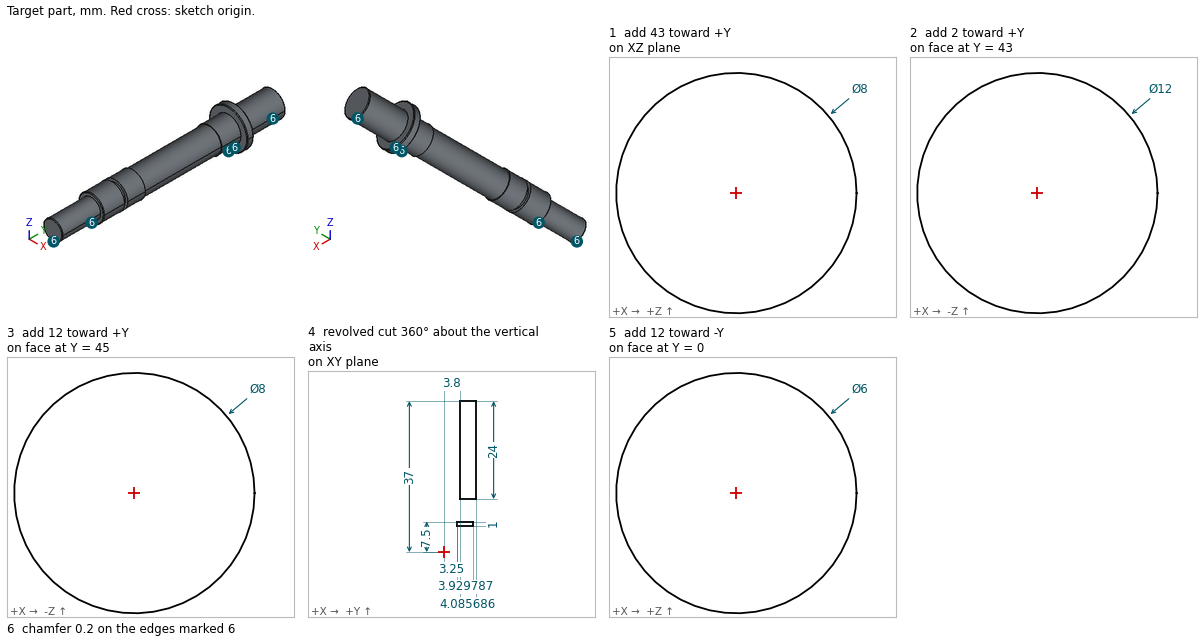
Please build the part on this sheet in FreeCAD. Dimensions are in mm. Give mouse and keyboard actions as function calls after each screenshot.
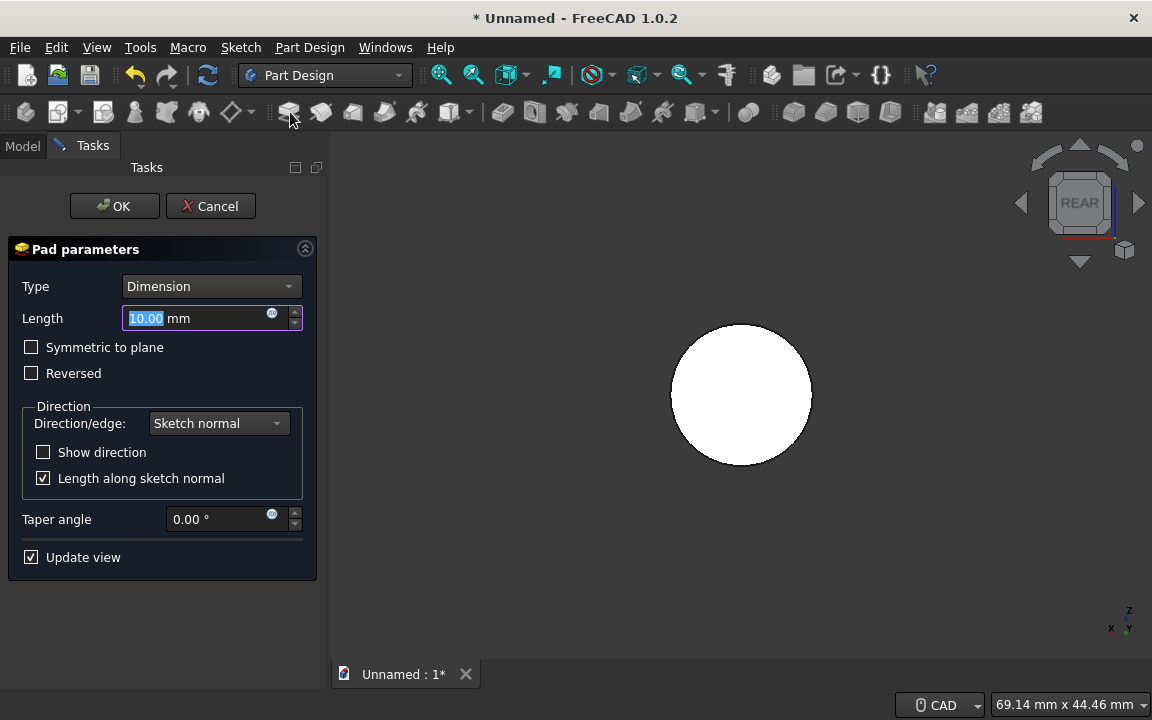
text(2)
key(Tab)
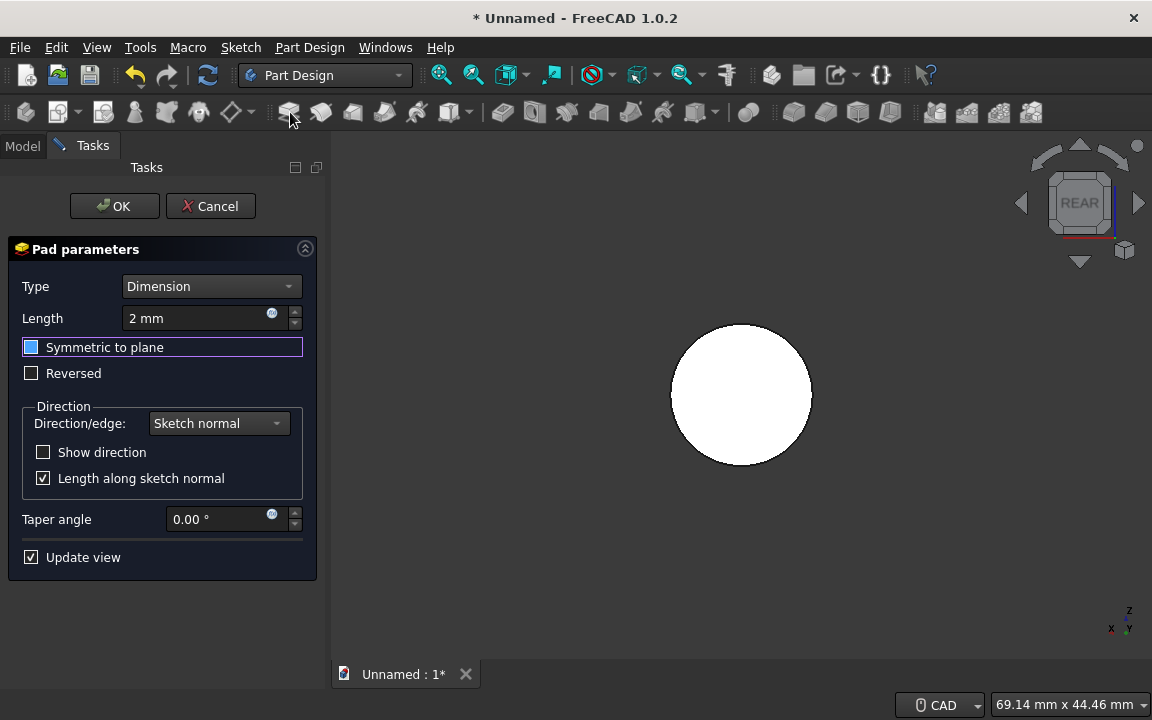
click(115, 206)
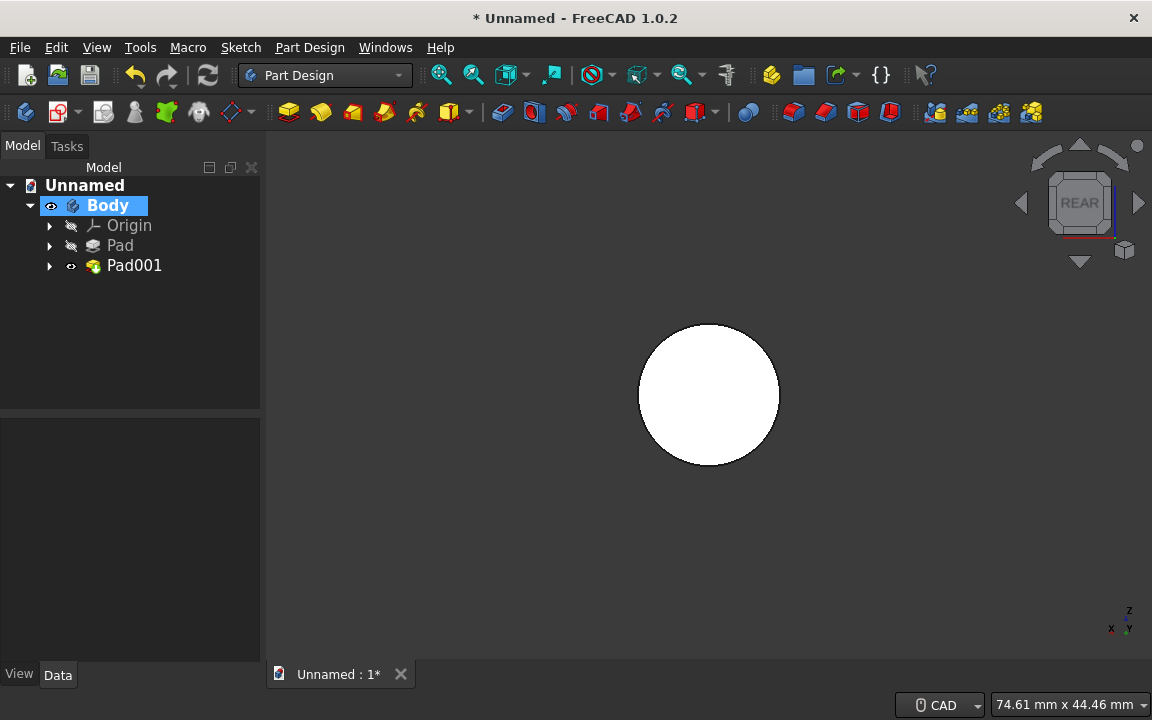
click(442, 76)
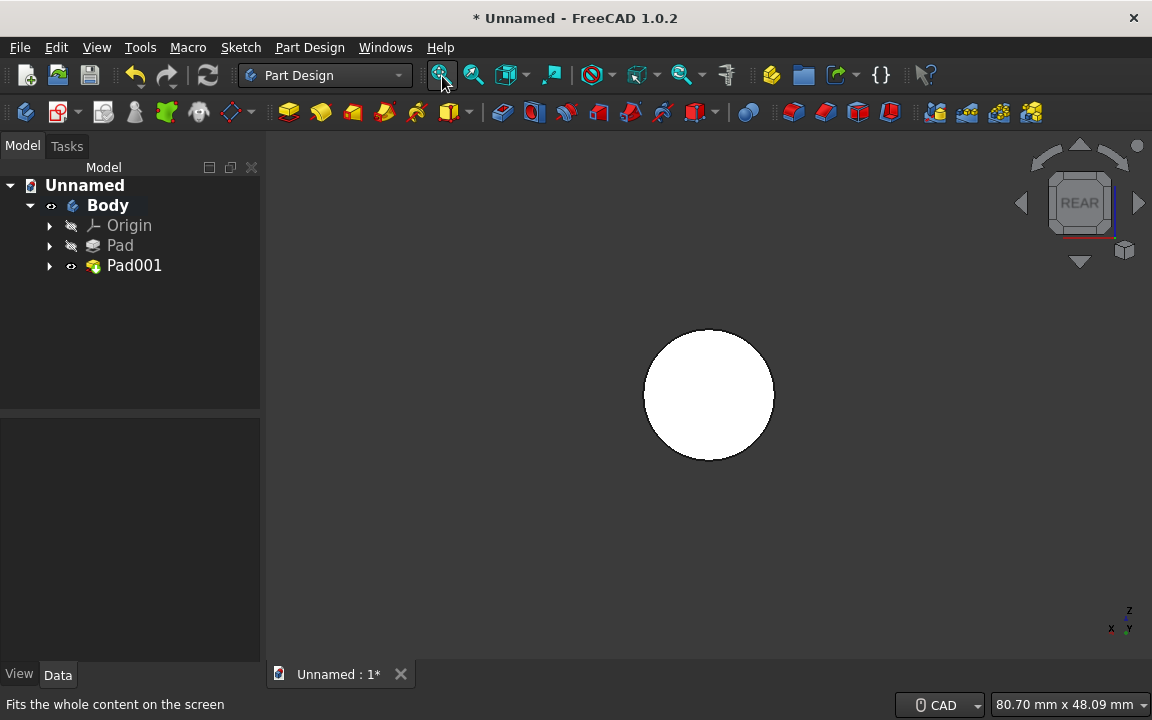
click(709, 394)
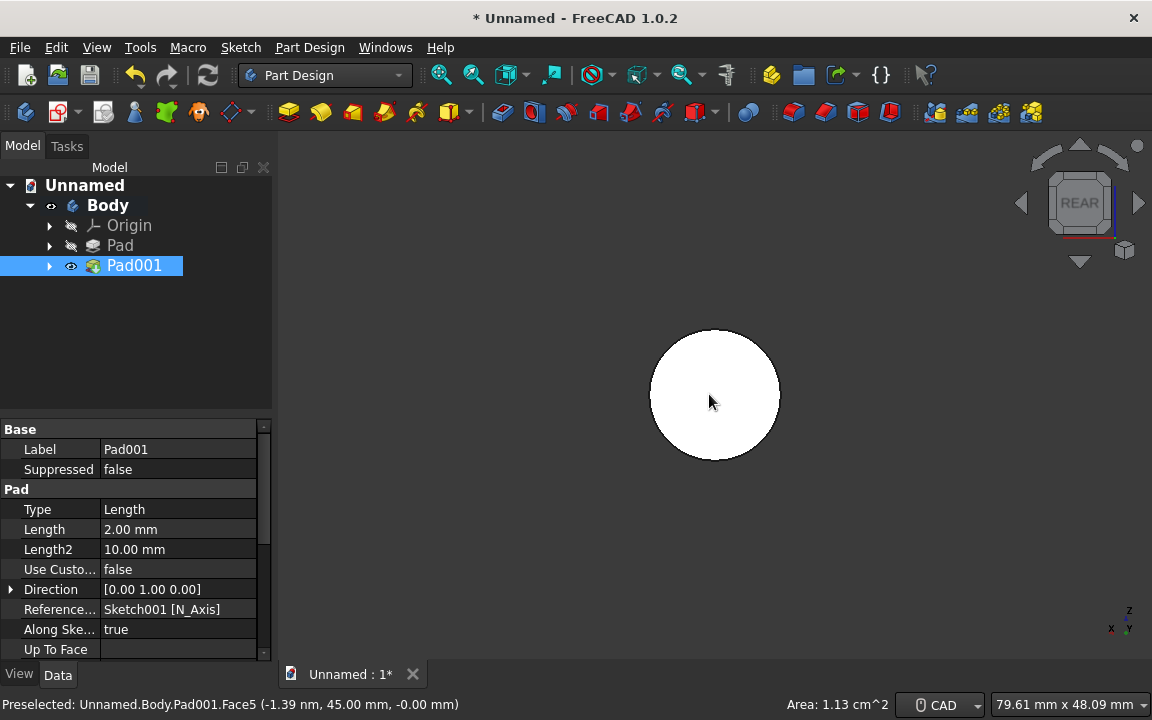
click(58, 112)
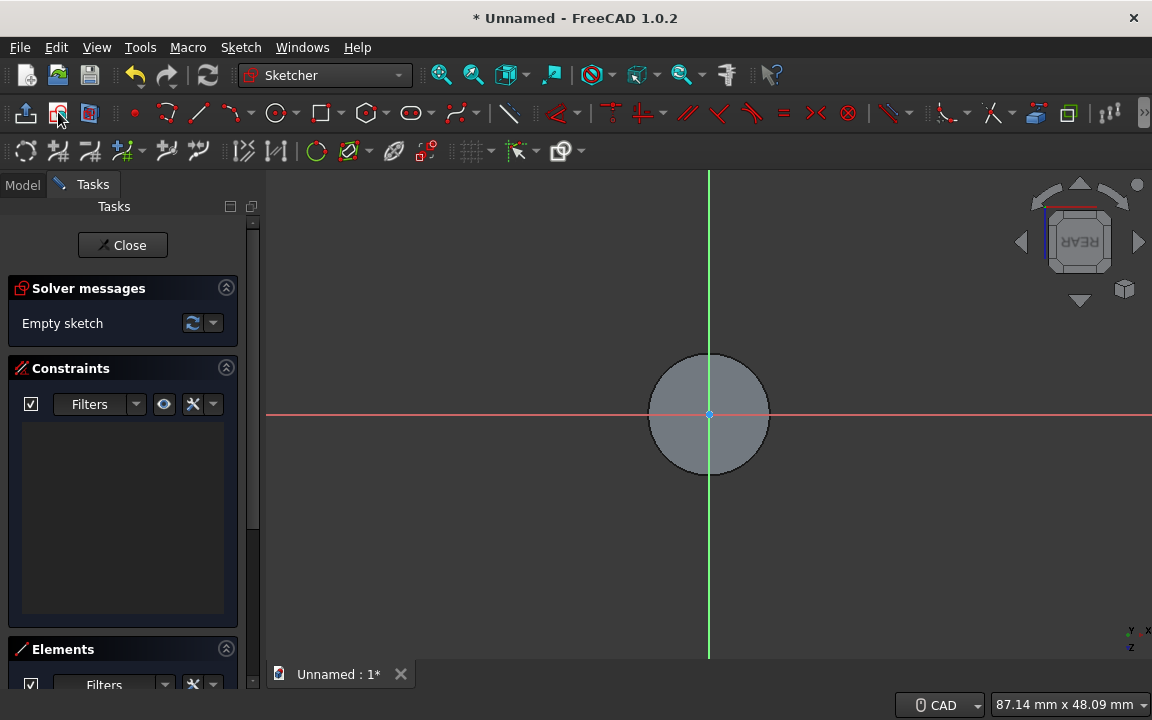
scroll(731, 414, up, 7)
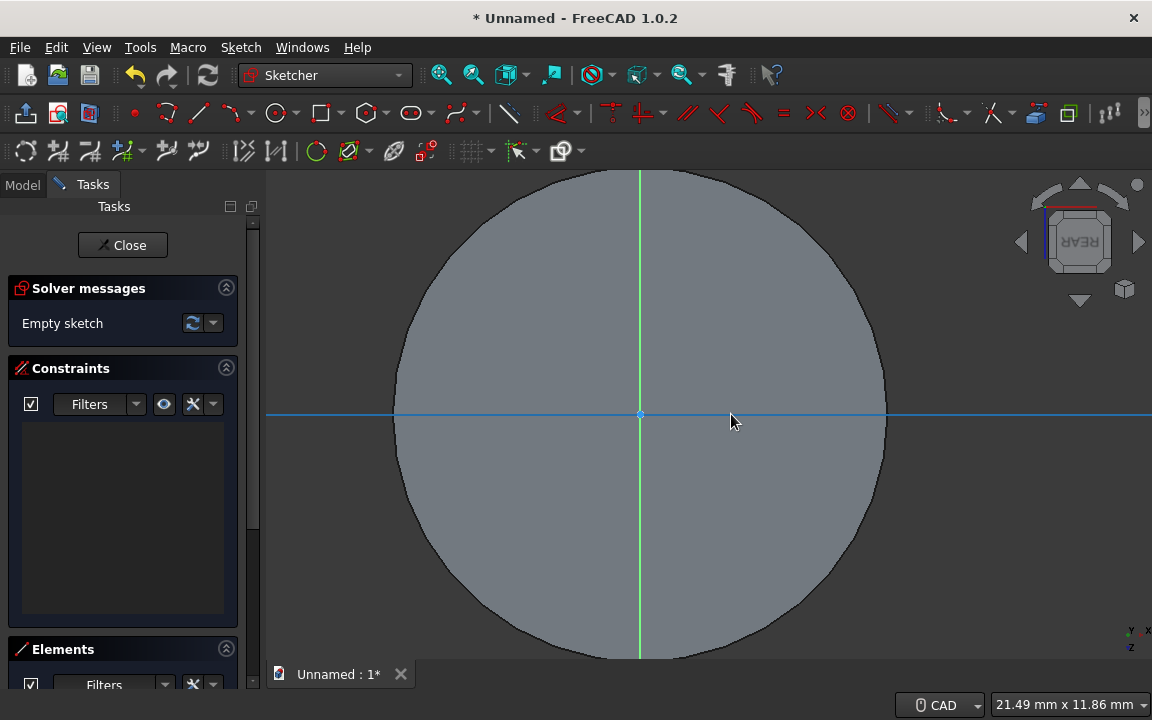
click(276, 114)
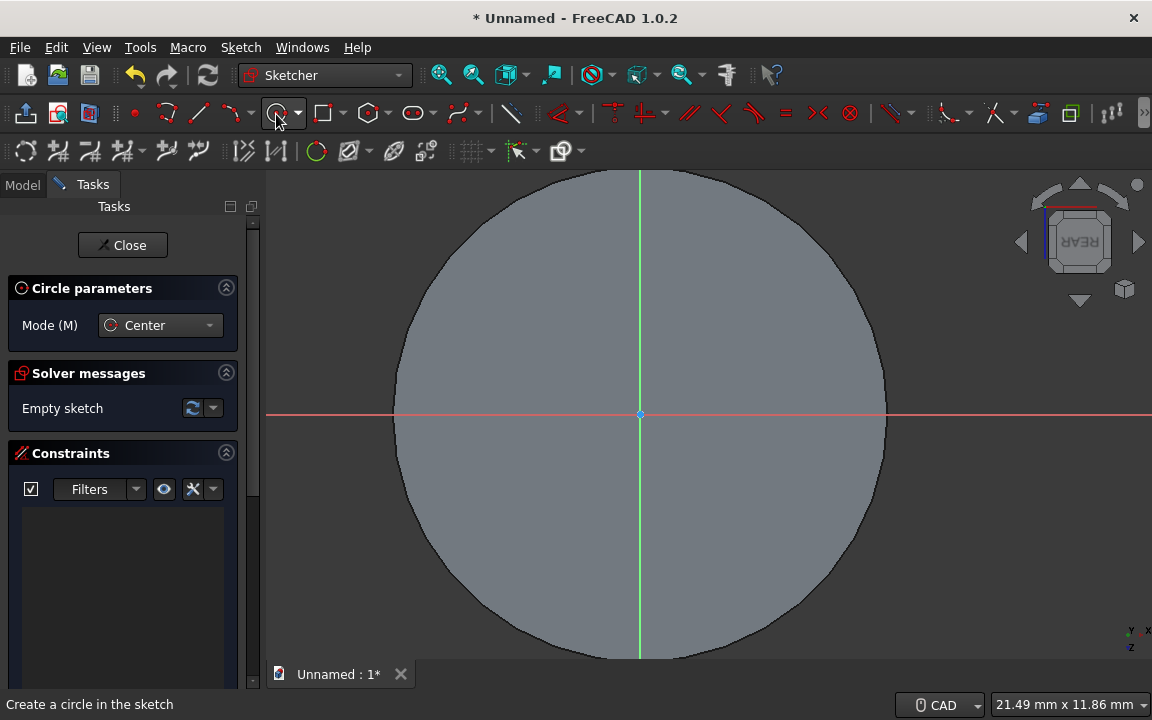
click(640, 414)
move(757, 298)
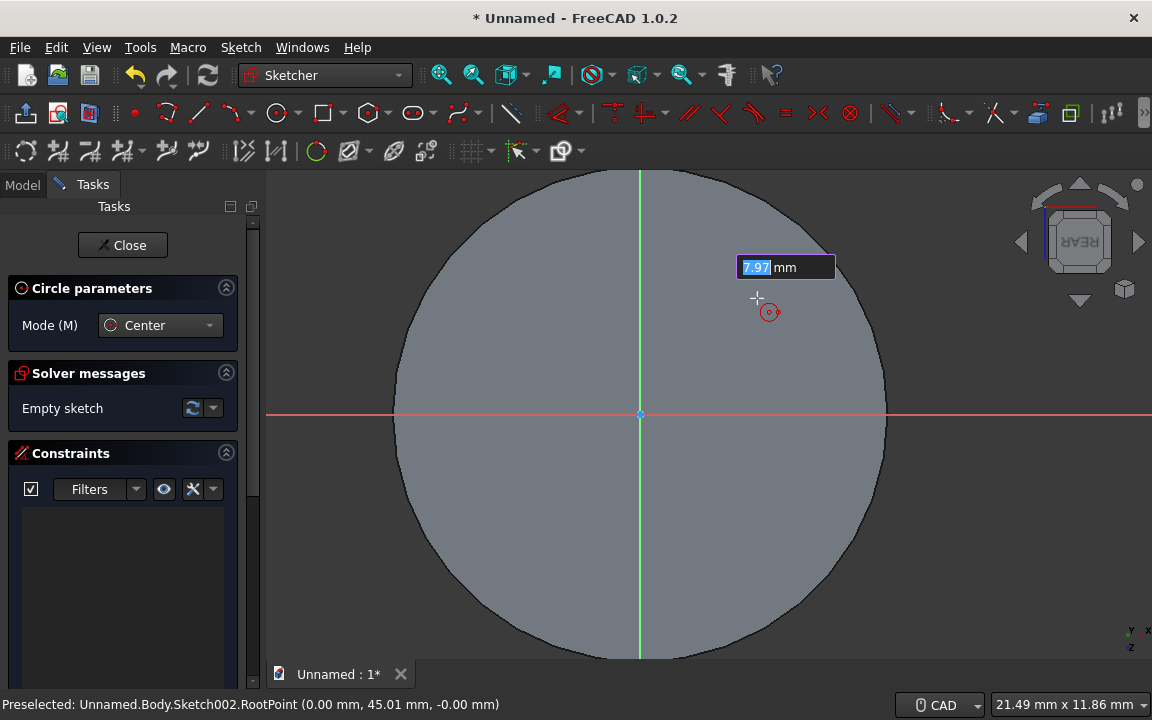
text(8)
key(Return)
key(Escape)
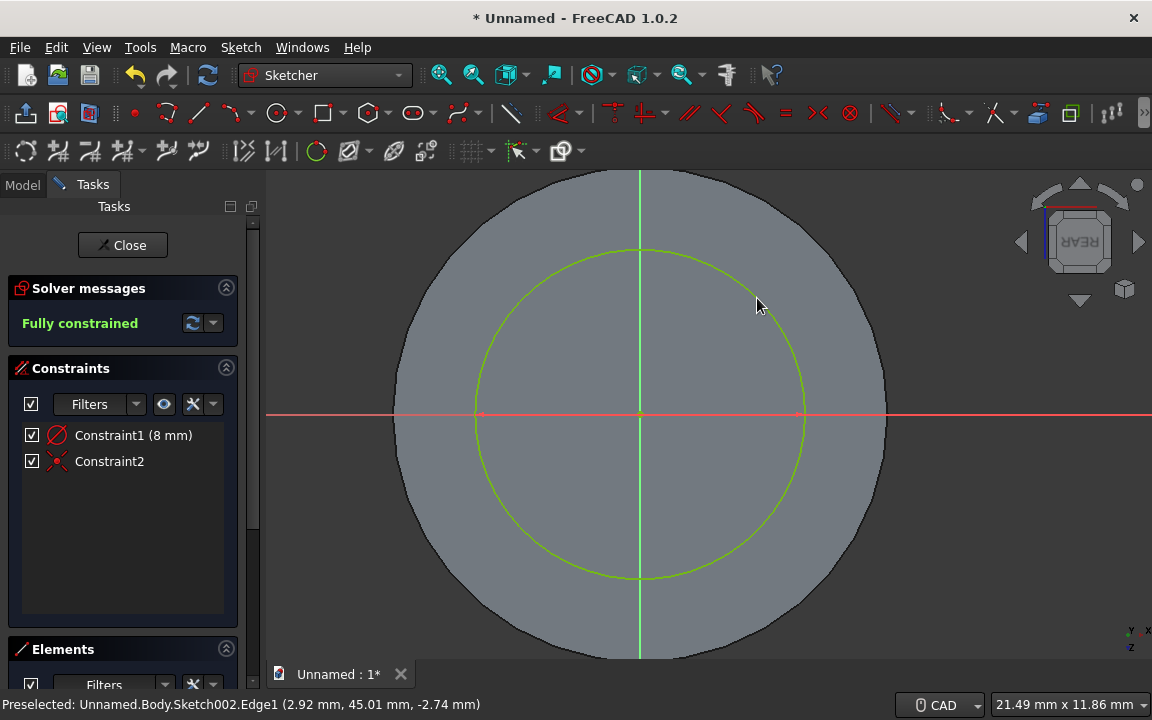
click(123, 245)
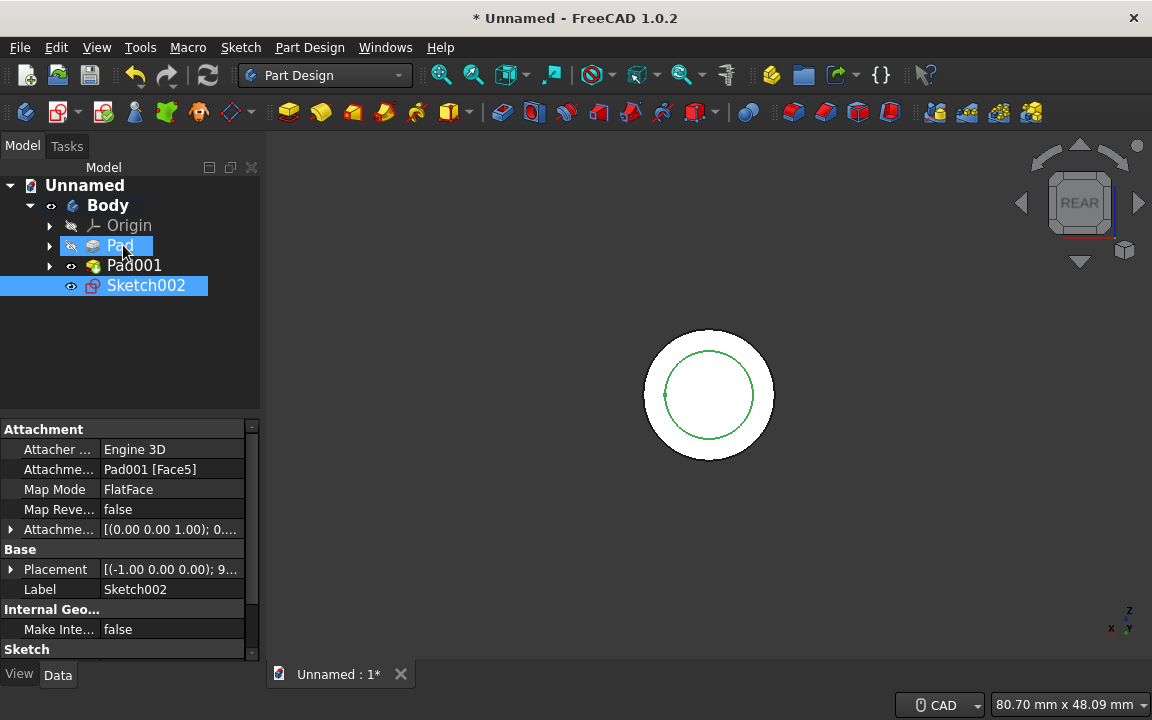
click(290, 112)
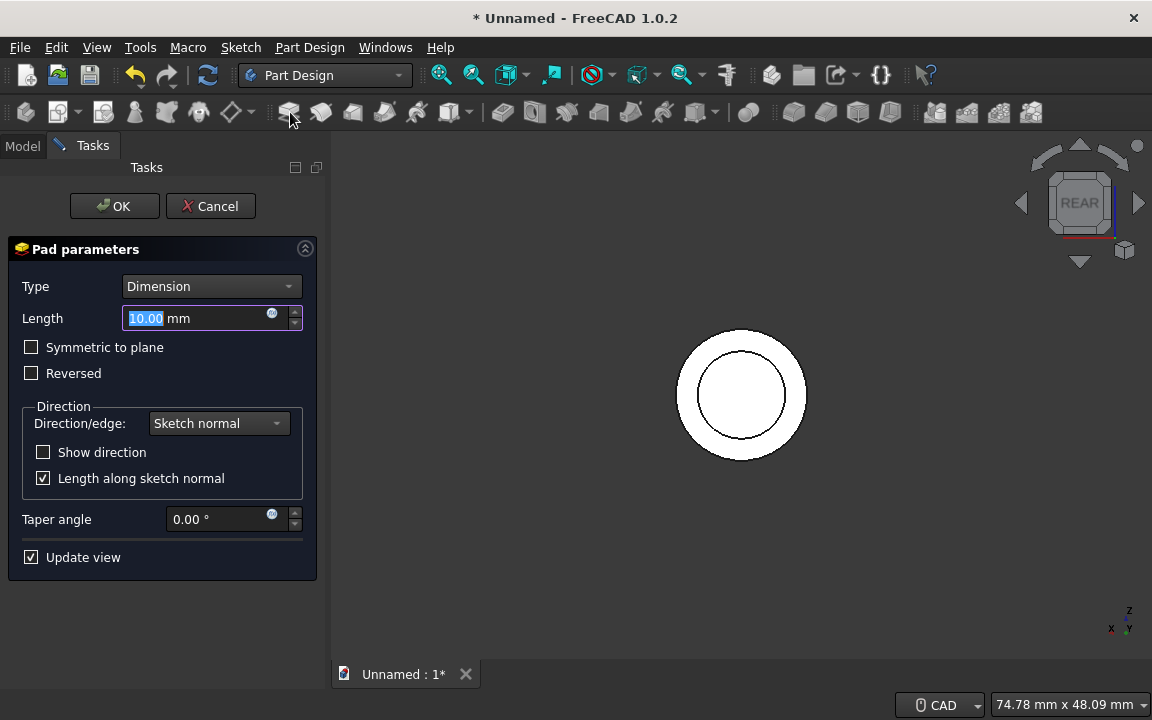
text(12)
key(Tab)